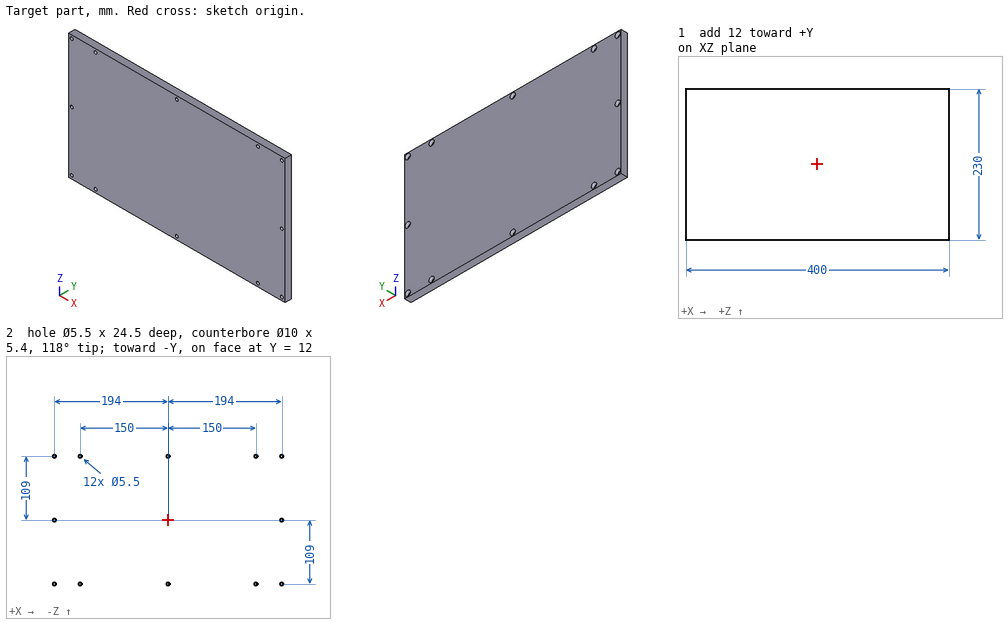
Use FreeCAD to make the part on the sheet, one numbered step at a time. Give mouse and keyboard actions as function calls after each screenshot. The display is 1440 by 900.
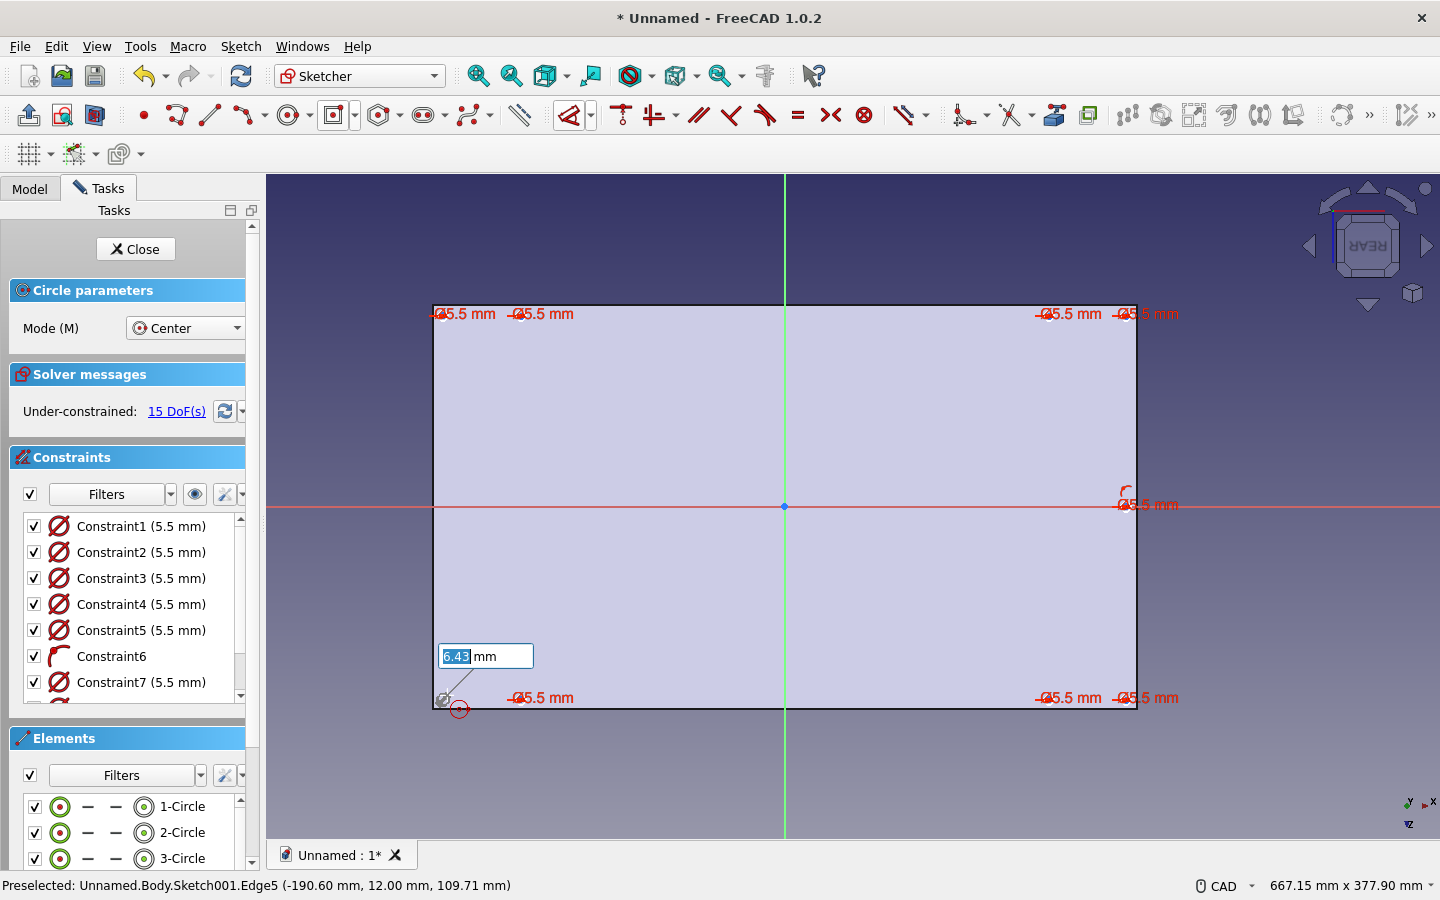
text(5.5)
key(Return)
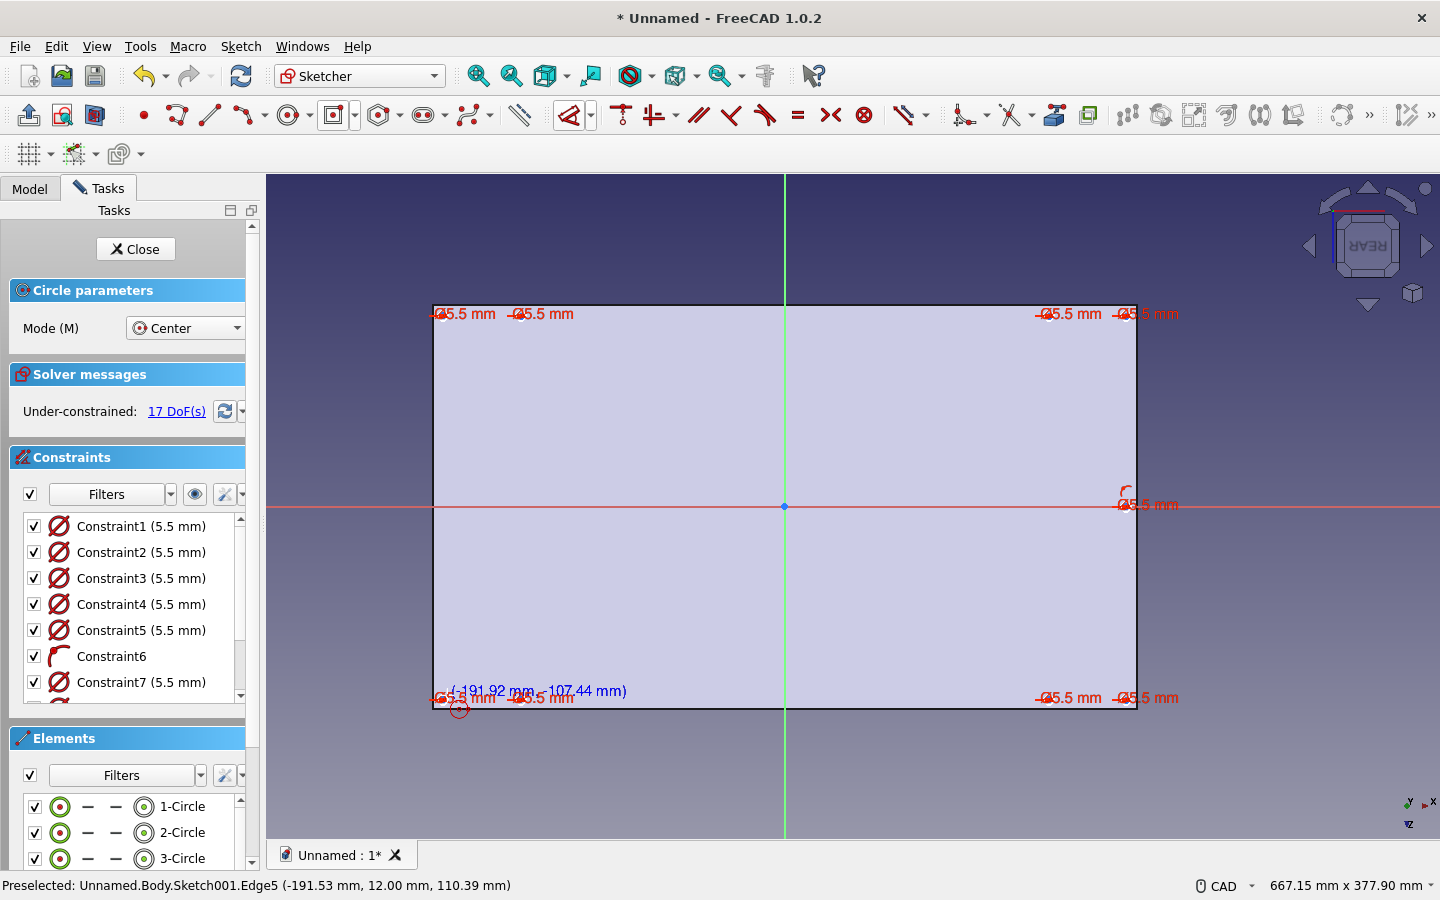
scroll(443, 507, up, 8)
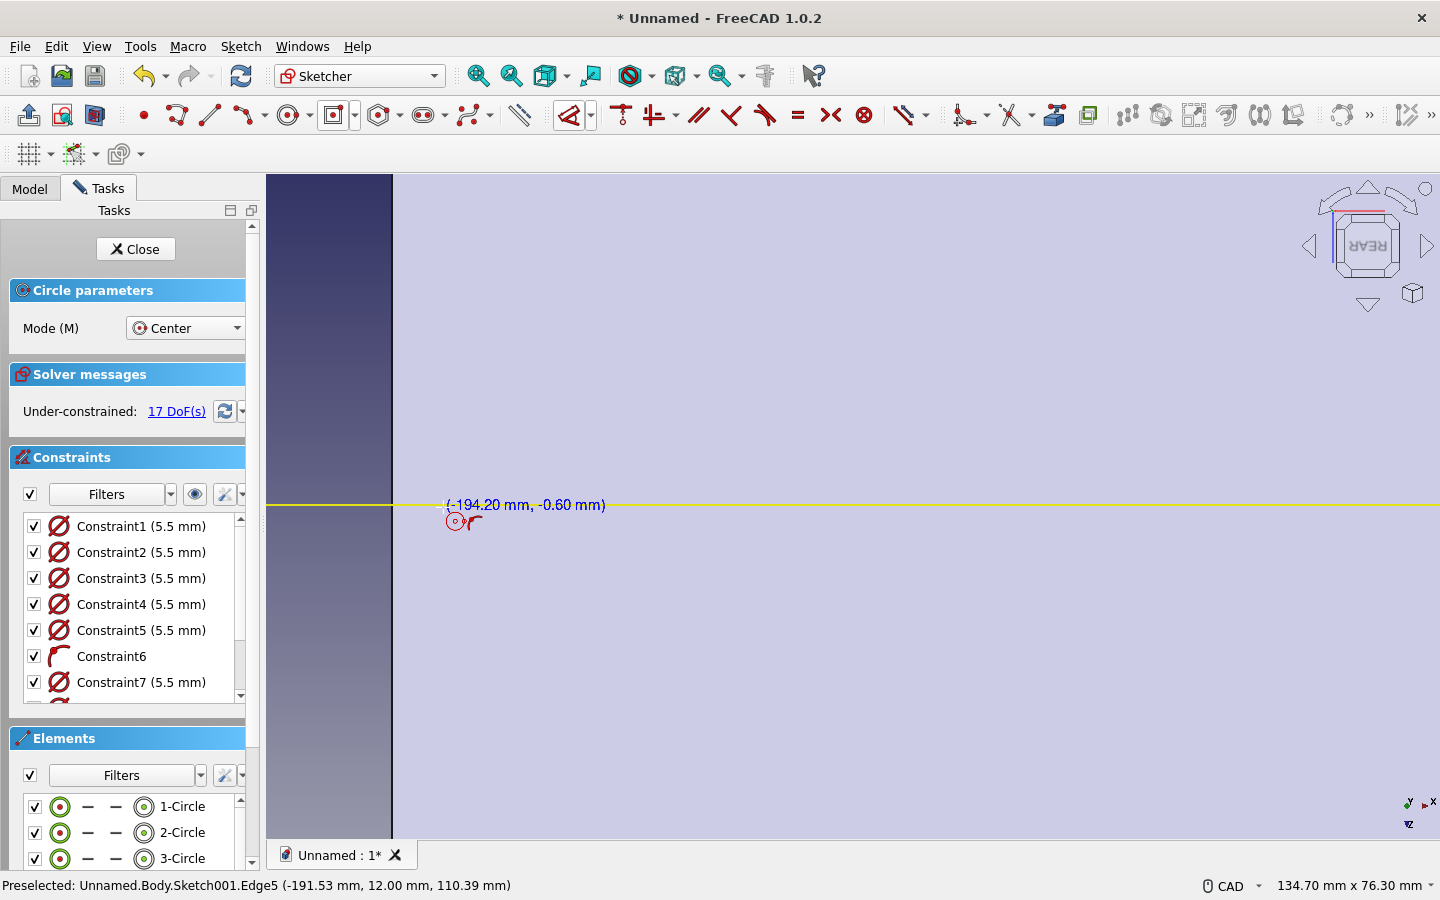
scroll(443, 507, down, 8)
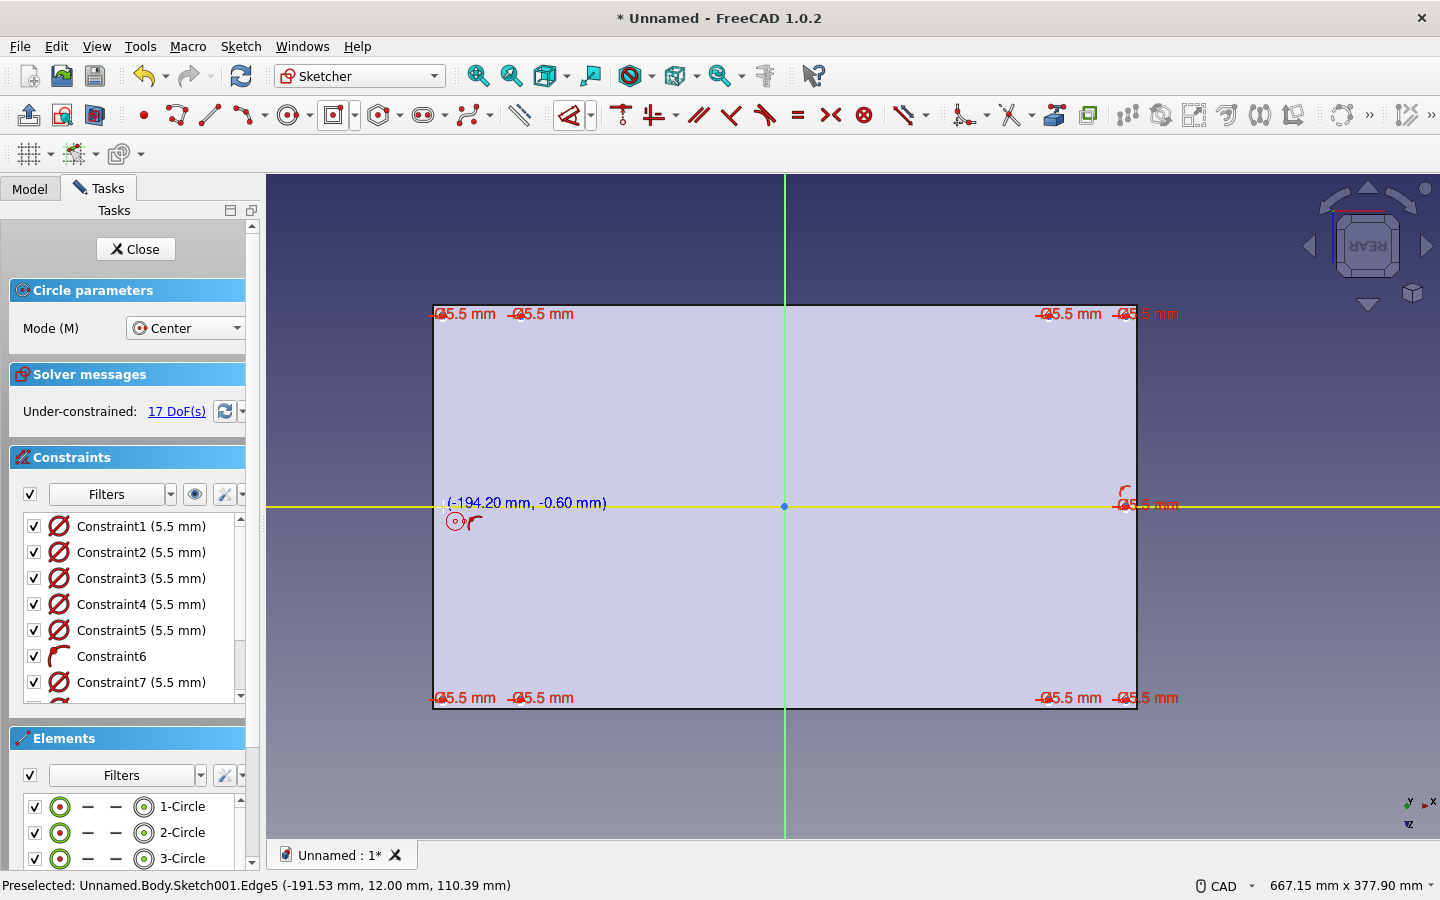
click(443, 507)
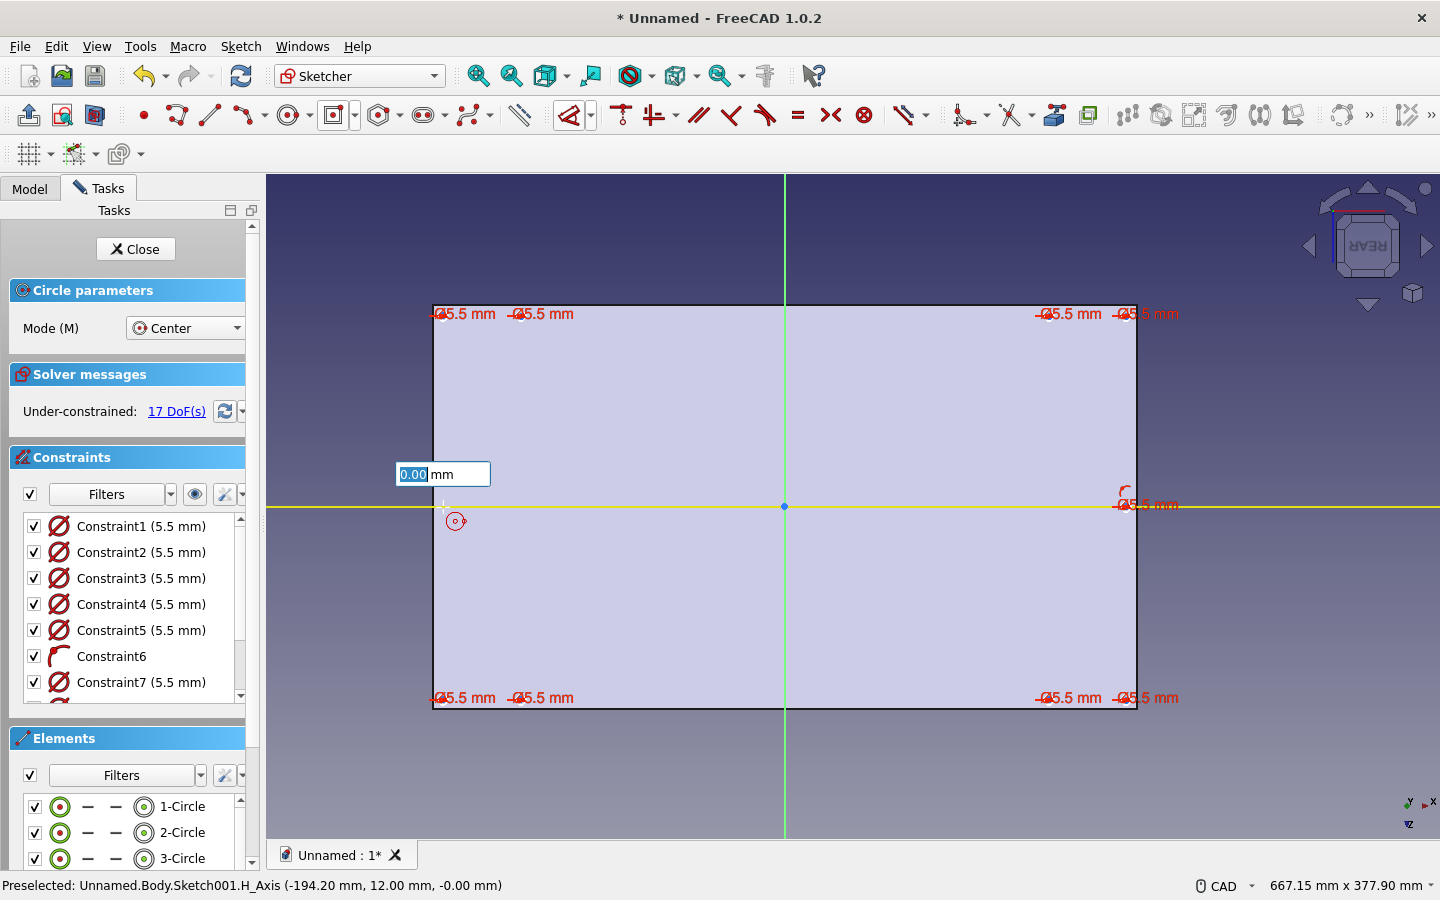
scroll(445, 502, up, 7)
move(445, 502)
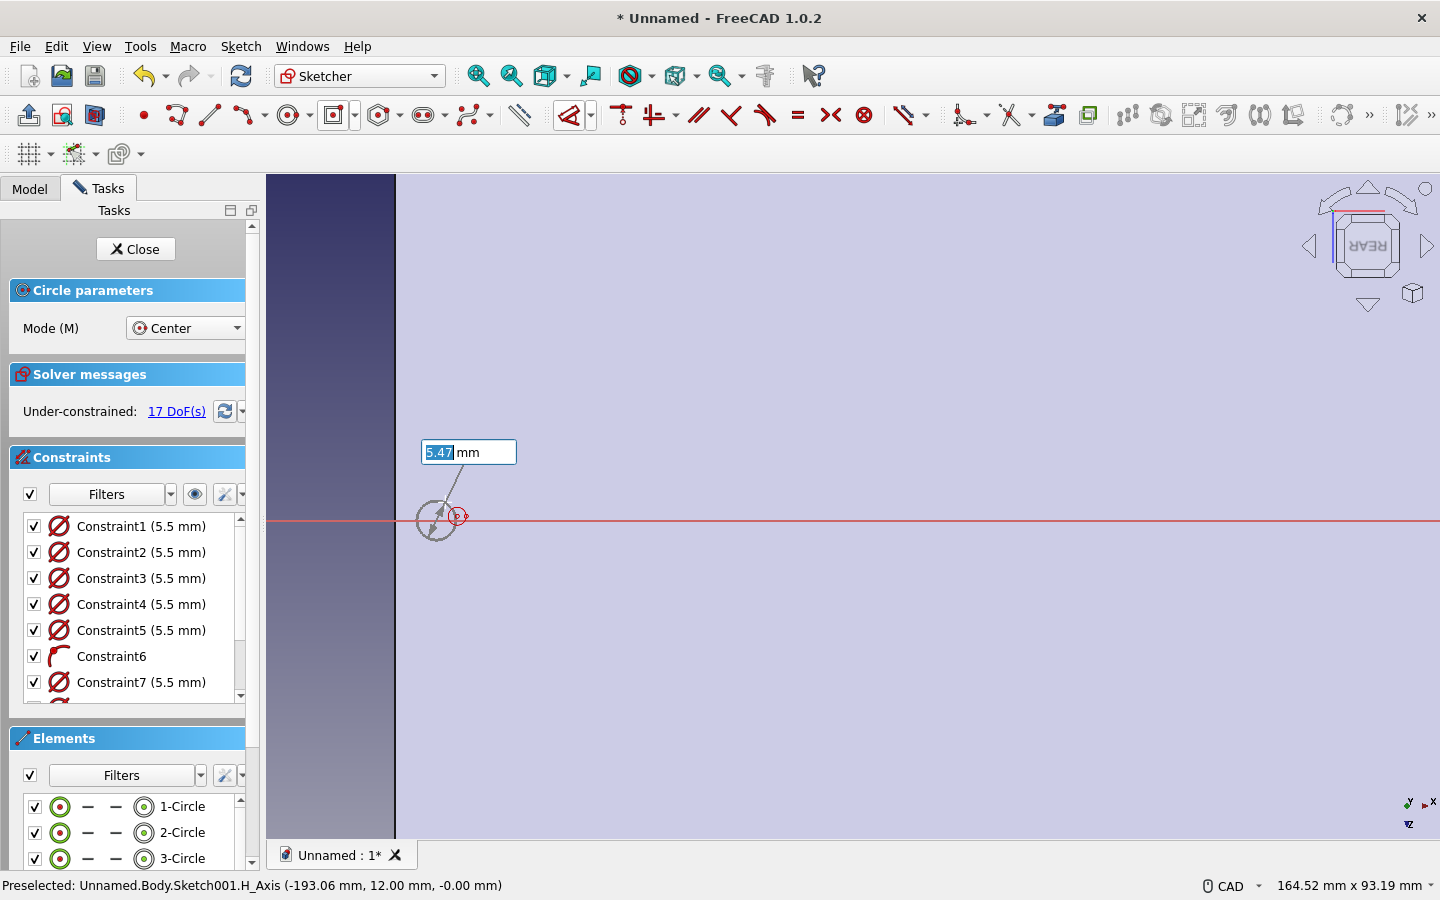
text(5.5)
key(Return)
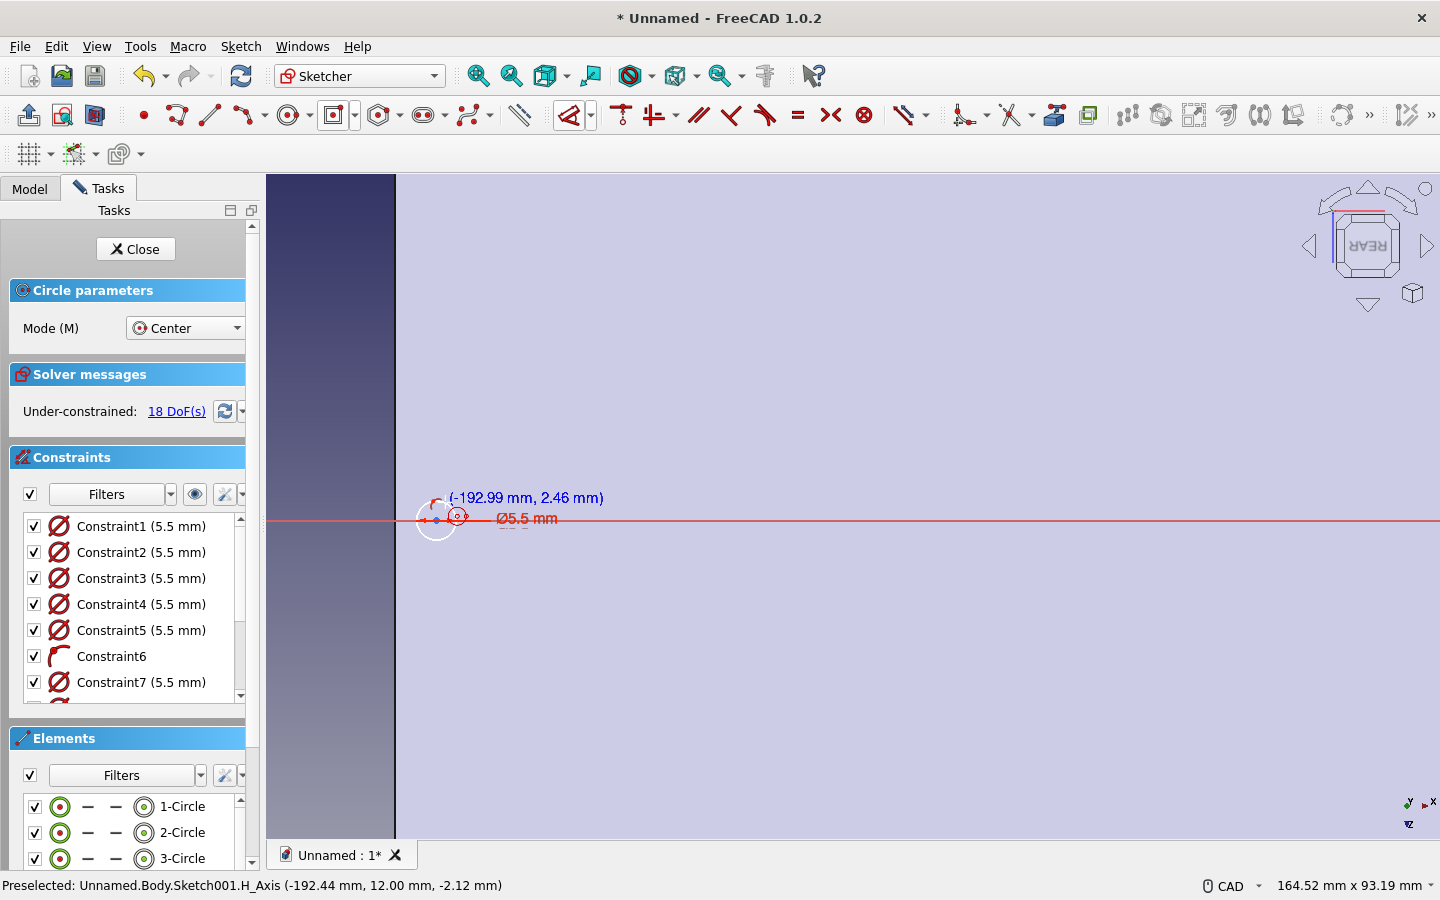
scroll(445, 502, down, 7)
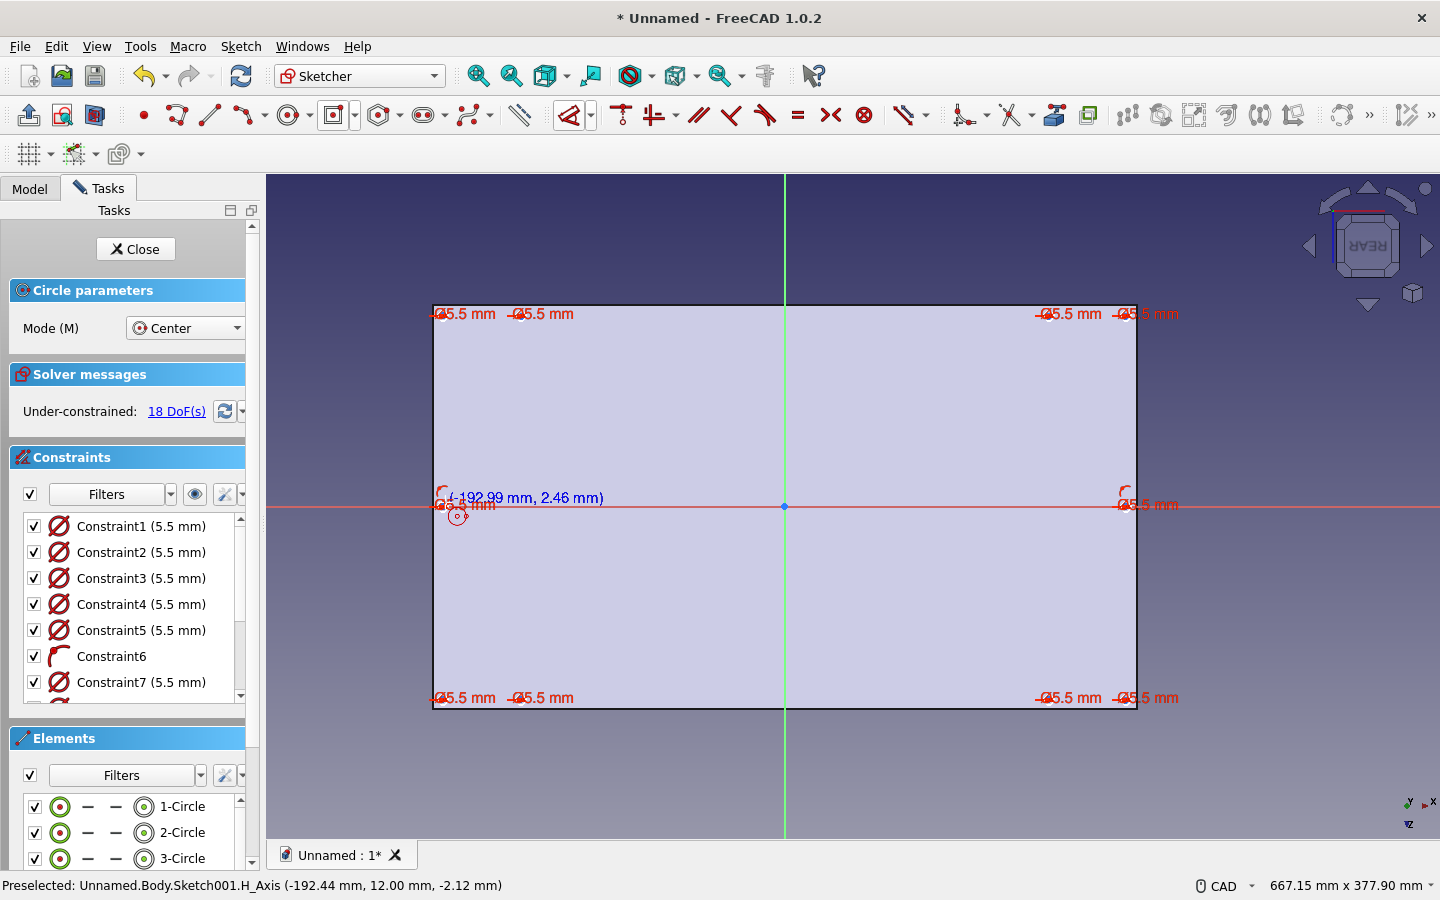
scroll(785, 315, up, 8)